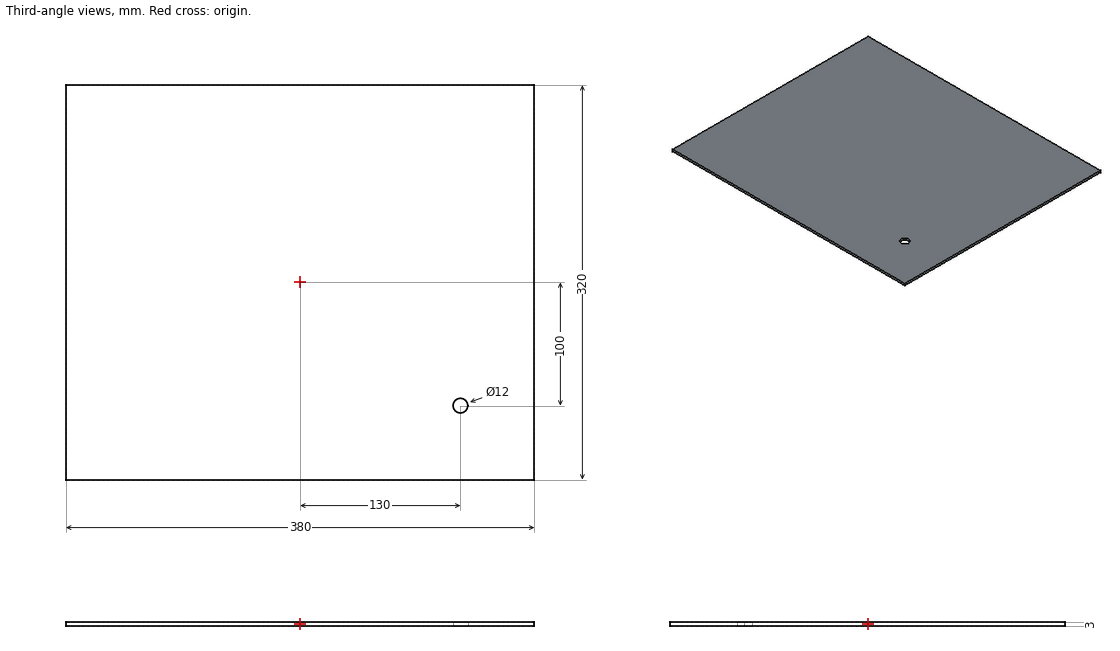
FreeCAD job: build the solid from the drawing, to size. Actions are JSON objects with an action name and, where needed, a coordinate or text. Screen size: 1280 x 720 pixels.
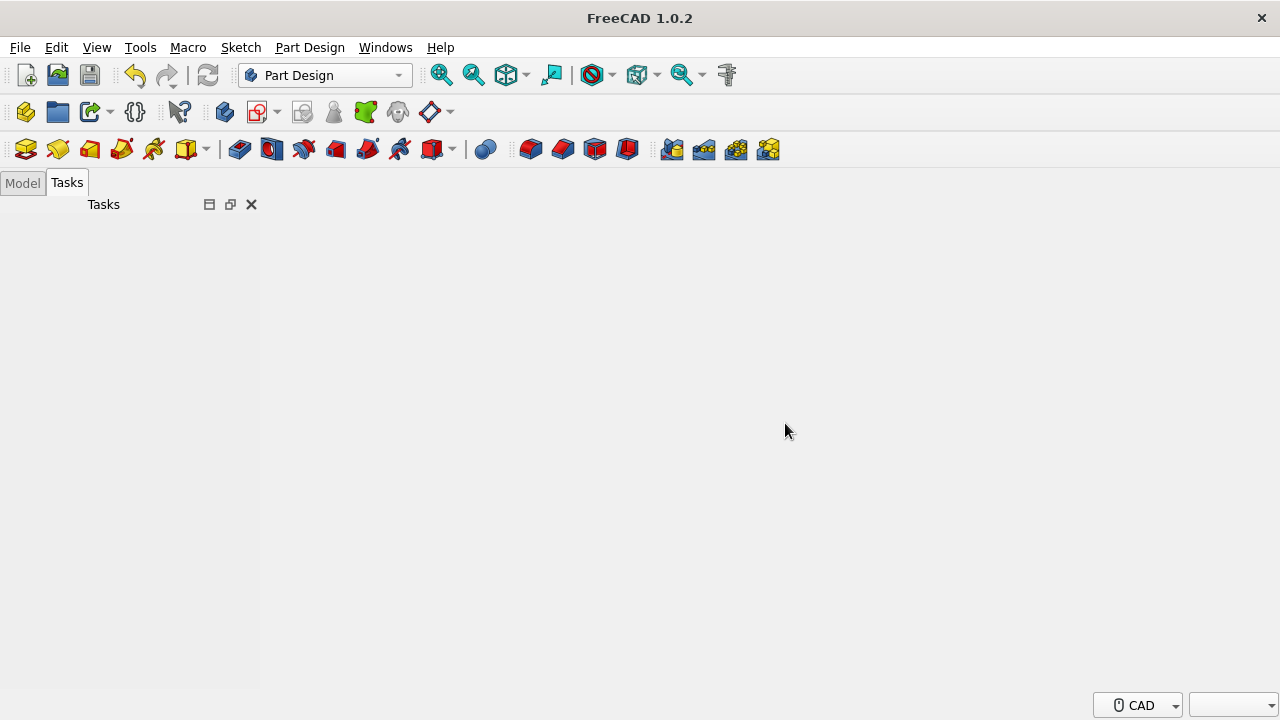
{"action": "left_click", "coordinate": [26, 76]}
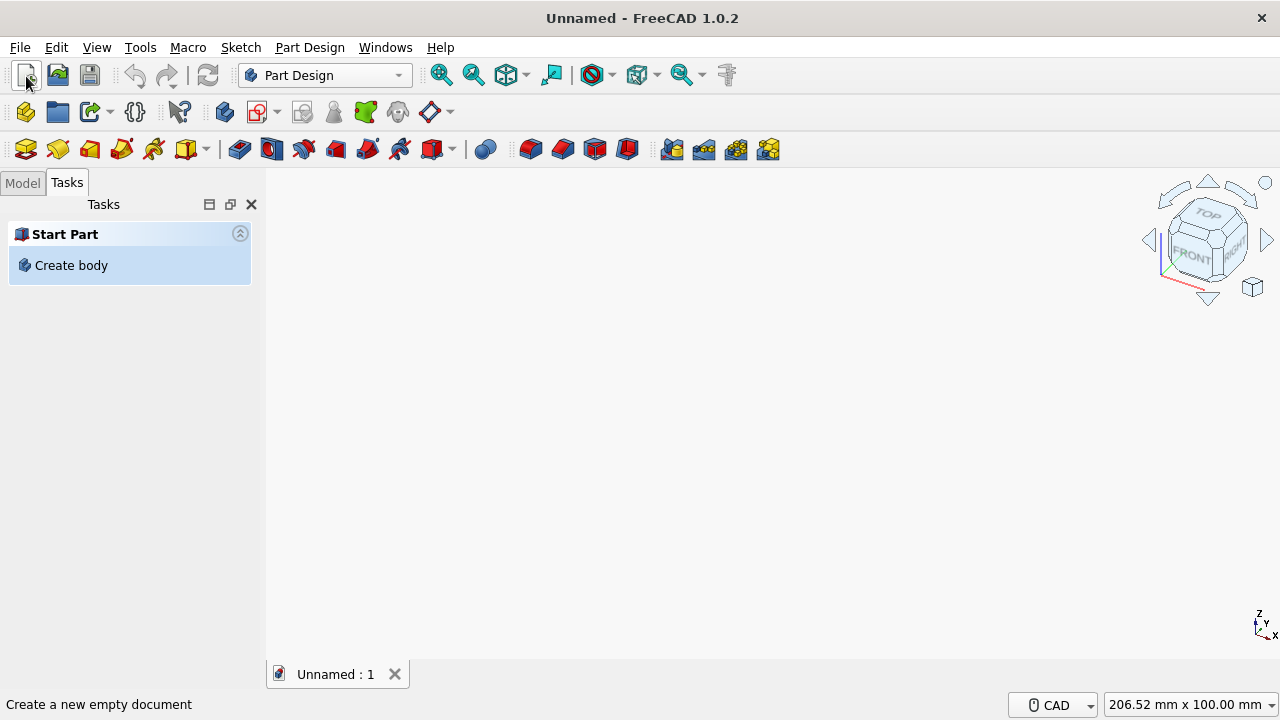
{"action": "left_click", "coordinate": [258, 112]}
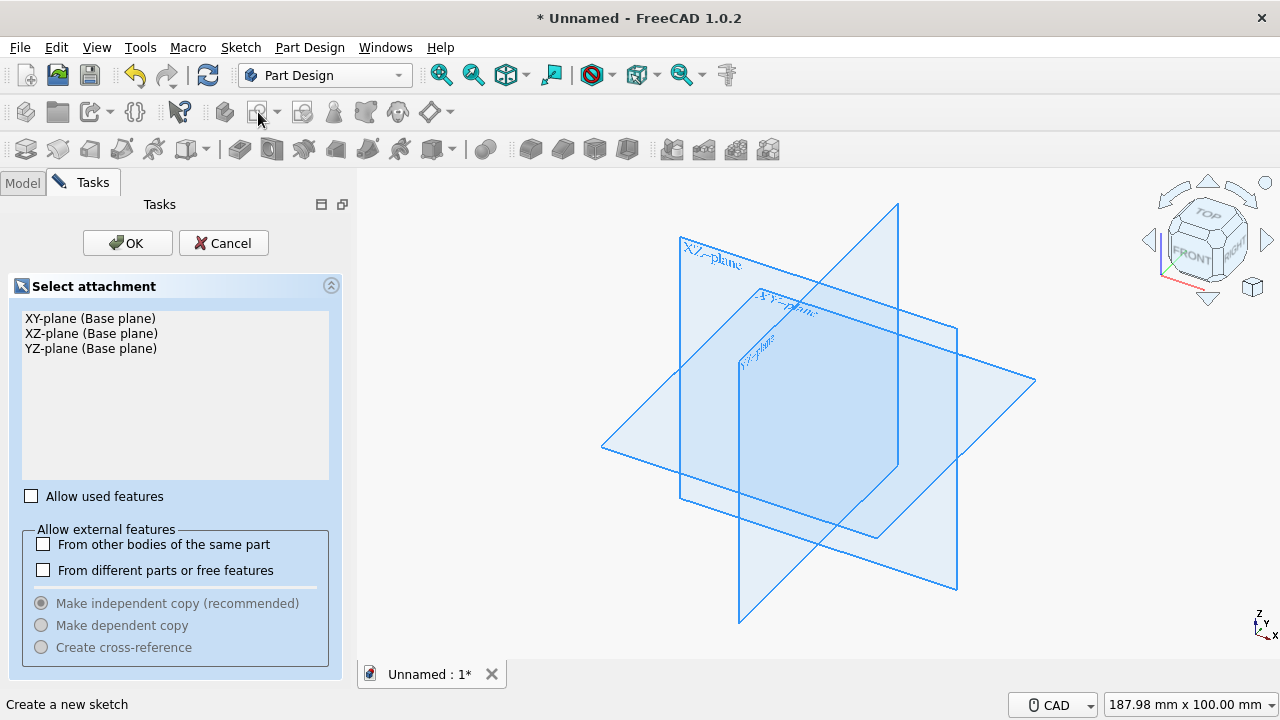
{"action": "left_click", "coordinate": [82, 318]}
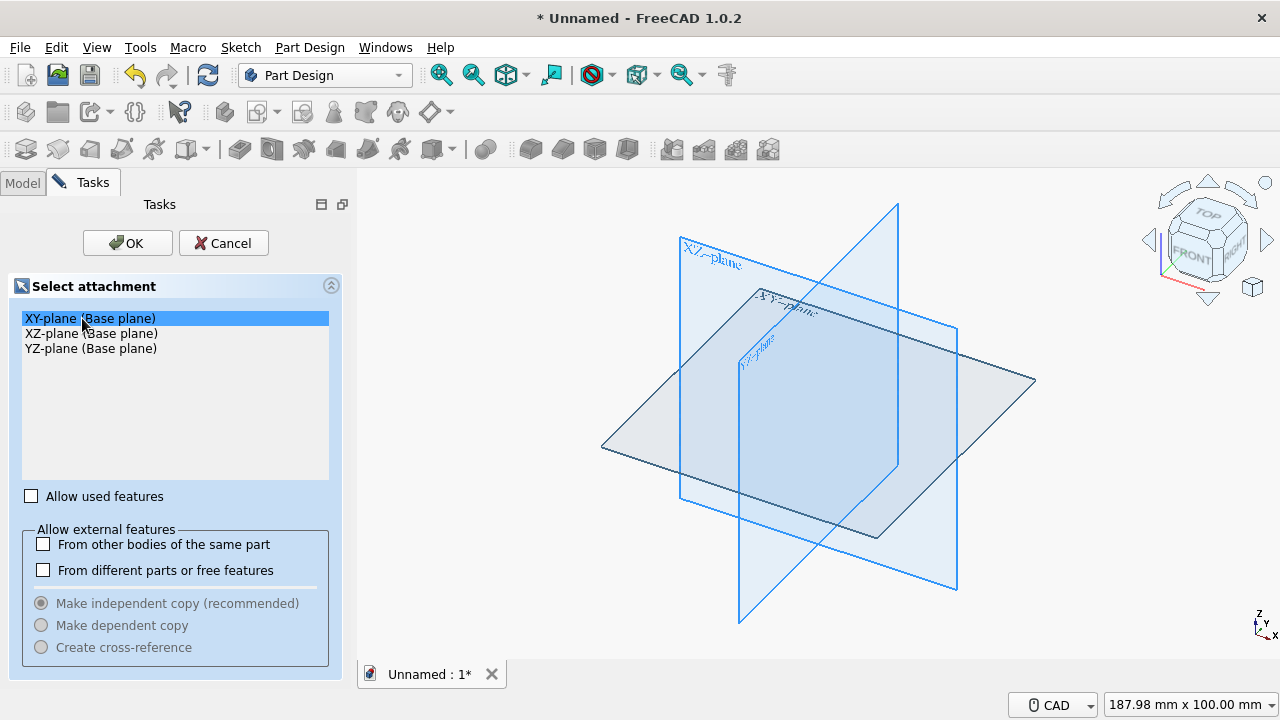
{"action": "left_click", "coordinate": [128, 243]}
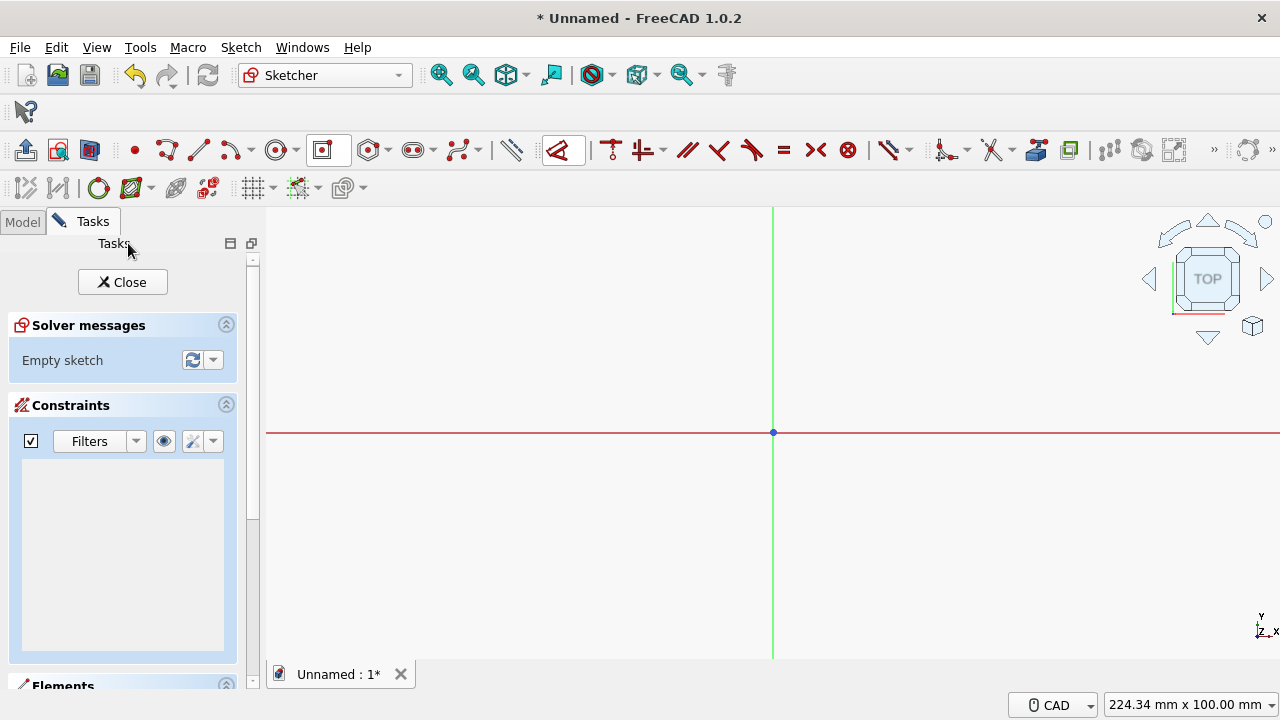
{"action": "scroll", "coordinate": [687, 433], "scroll_direction": "down", "scroll_amount": 8}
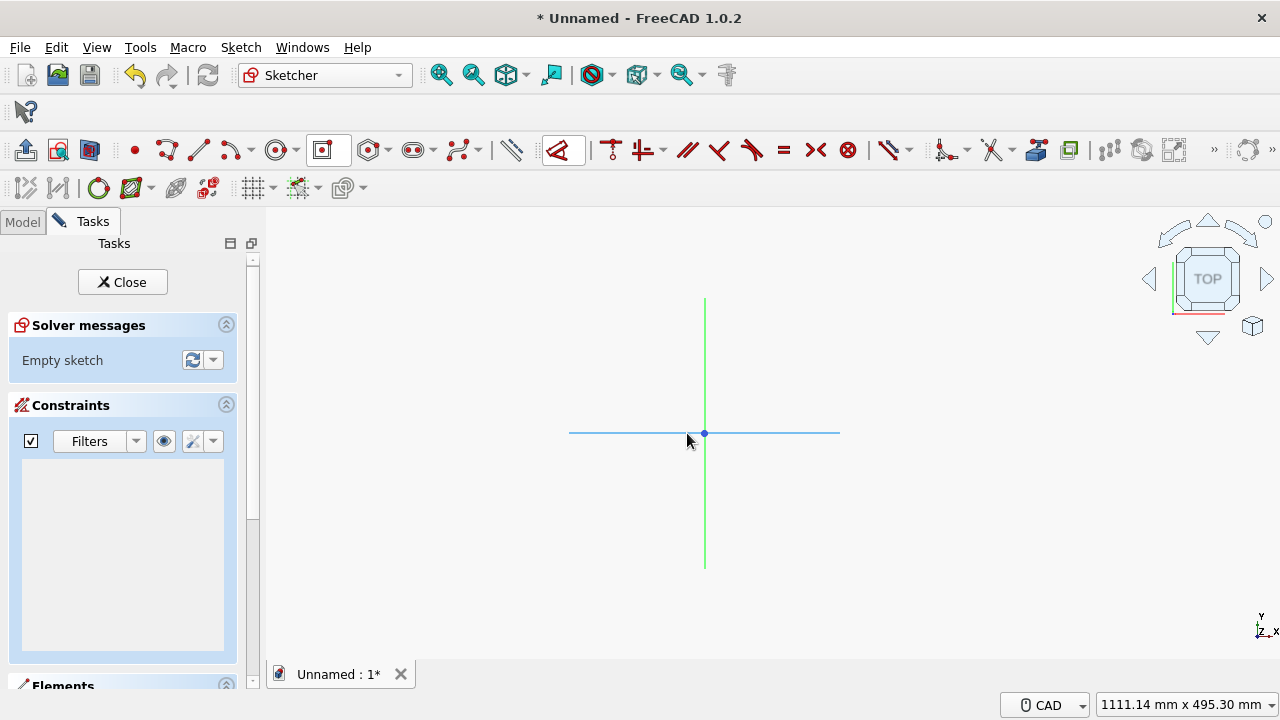
{"action": "left_click", "coordinate": [322, 150]}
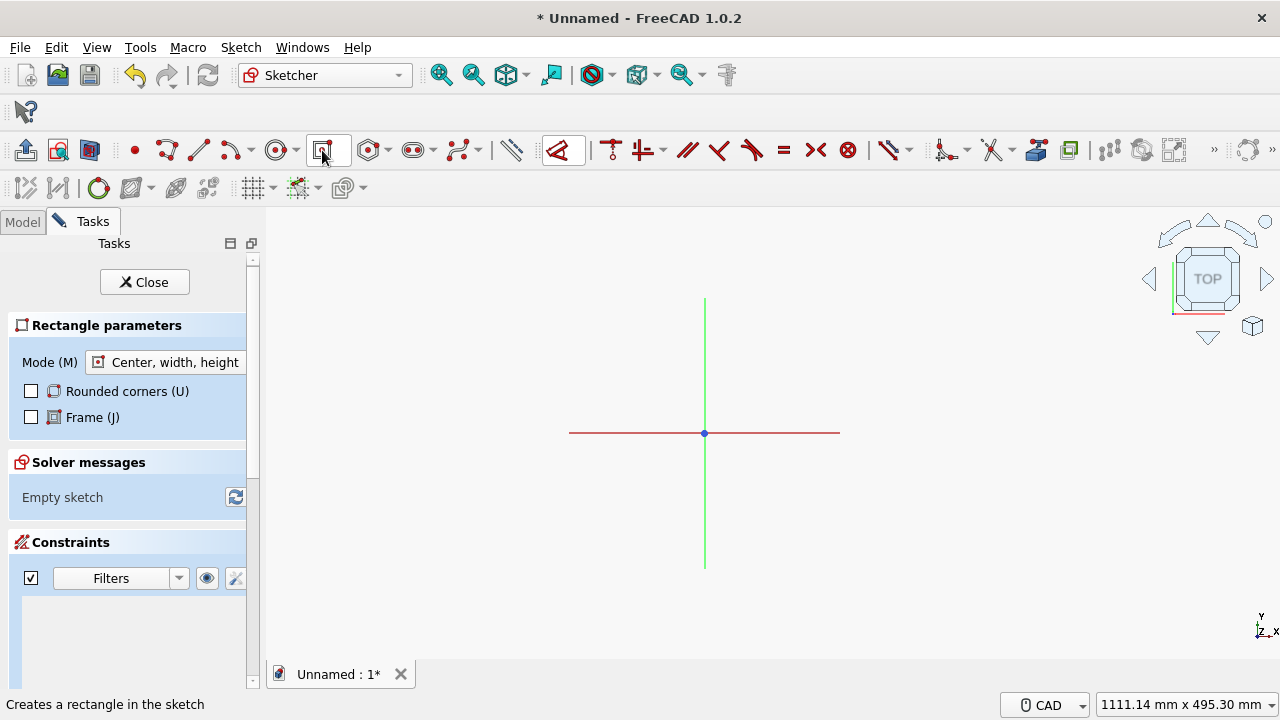
{"action": "left_click", "coordinate": [705, 433]}
{"action": "mouse_move", "coordinate": [878, 287]}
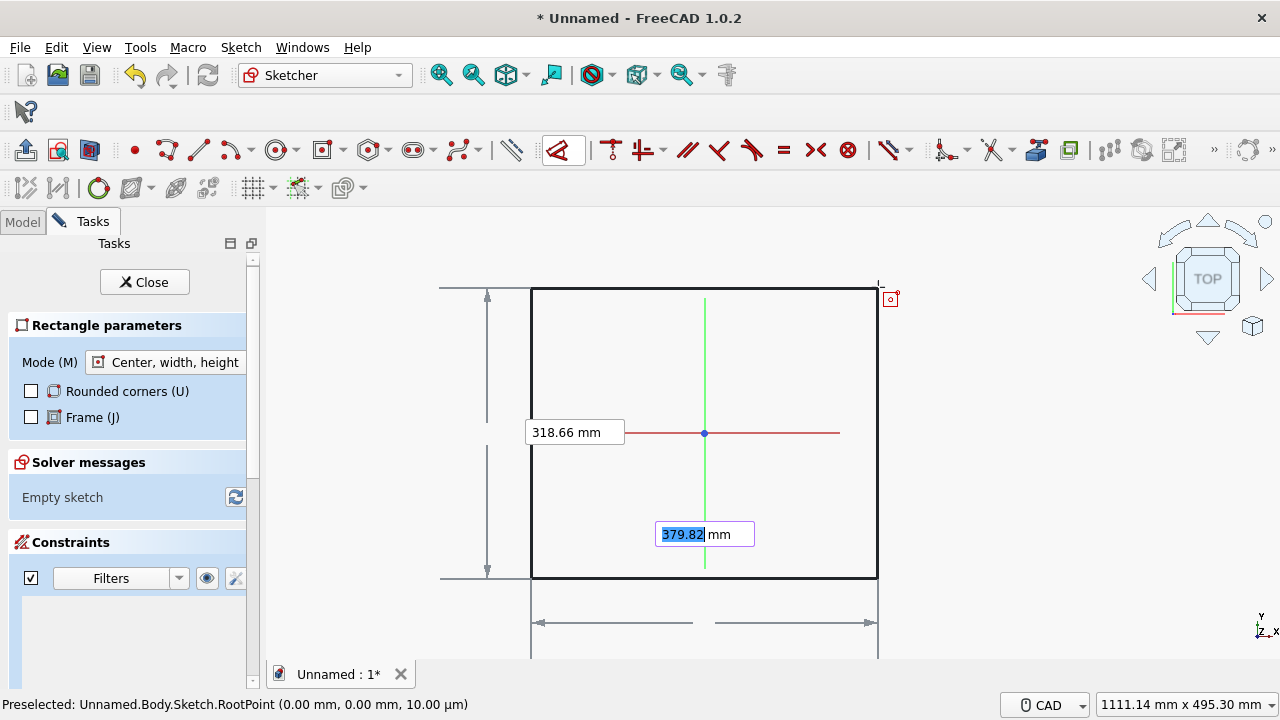
{"action": "type", "text": "380"}
{"action": "key", "text": "Tab"}
{"action": "type", "text": "320"}
{"action": "key", "text": "Return"}
{"action": "key", "text": "Escape"}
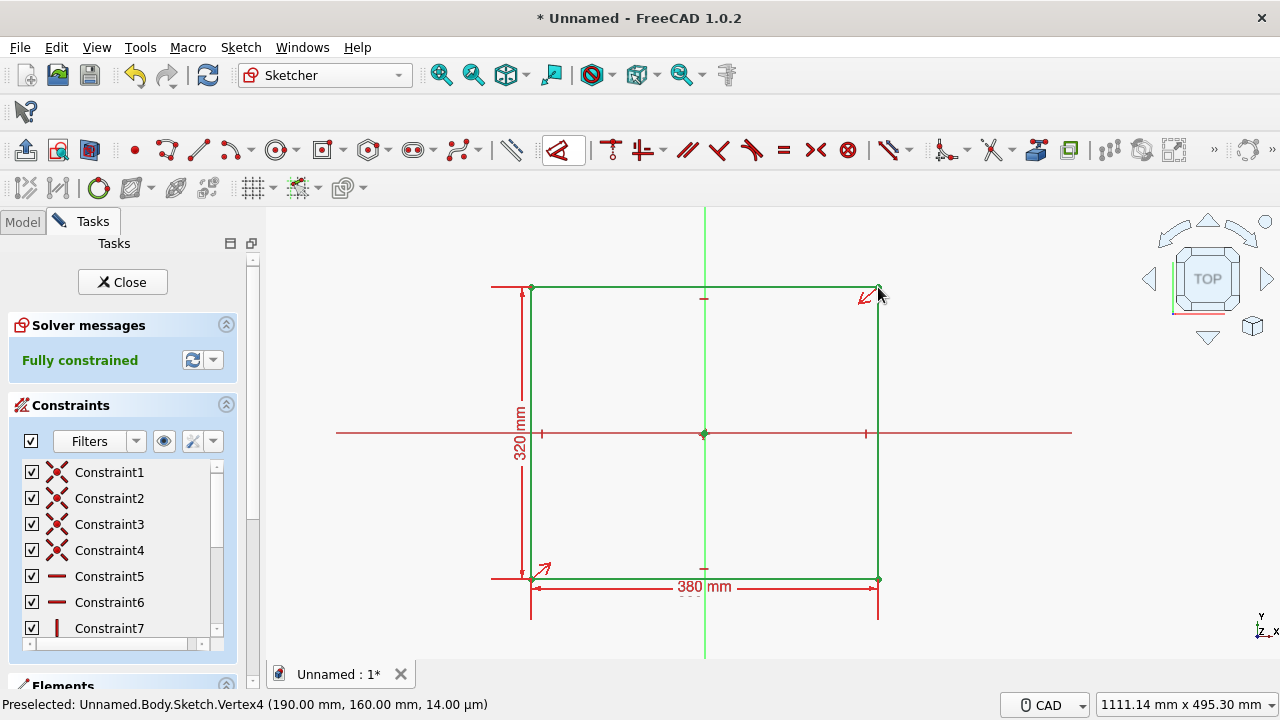
{"action": "left_click", "coordinate": [123, 282]}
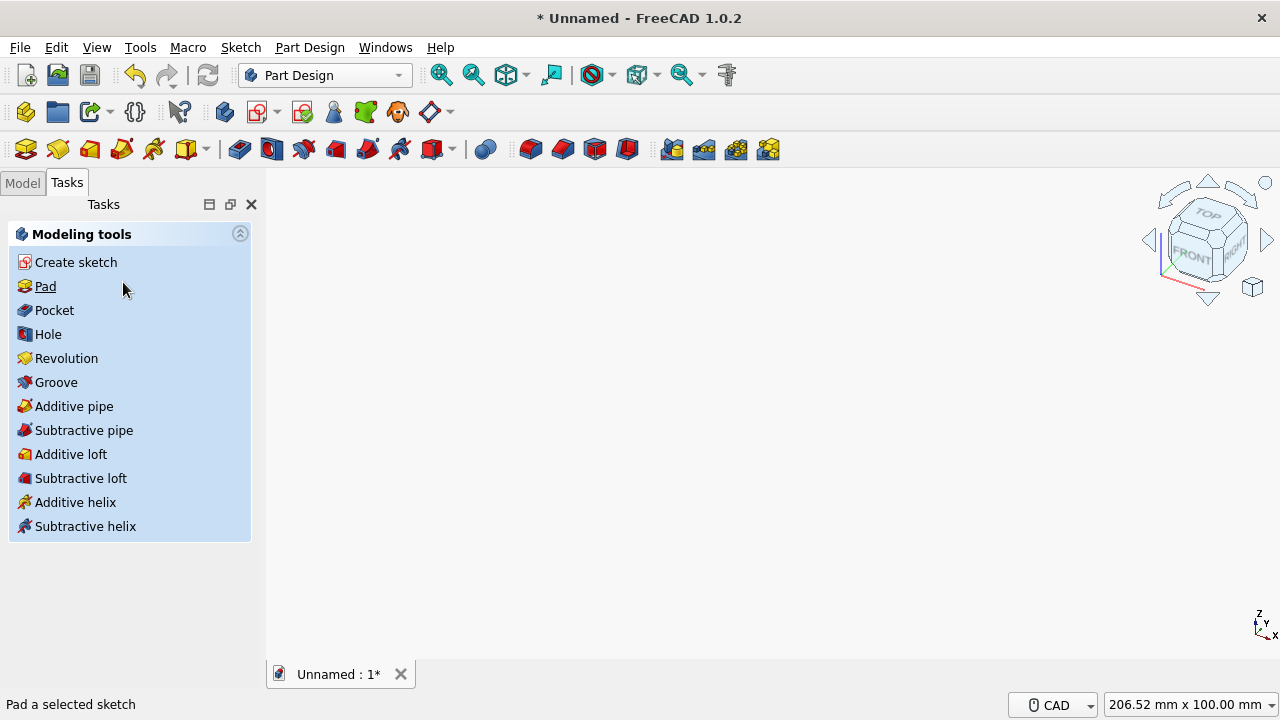
{"action": "left_click", "coordinate": [26, 150]}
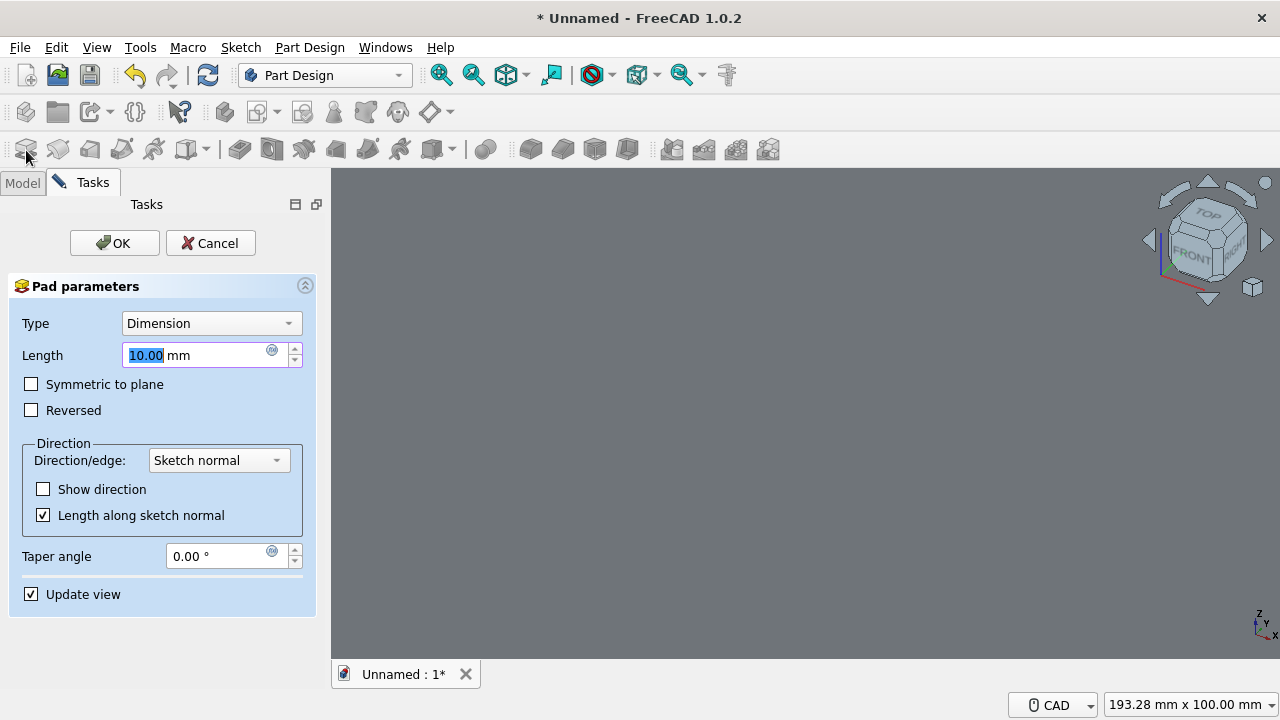
{"action": "type", "text": "3"}
{"action": "key", "text": "Tab"}